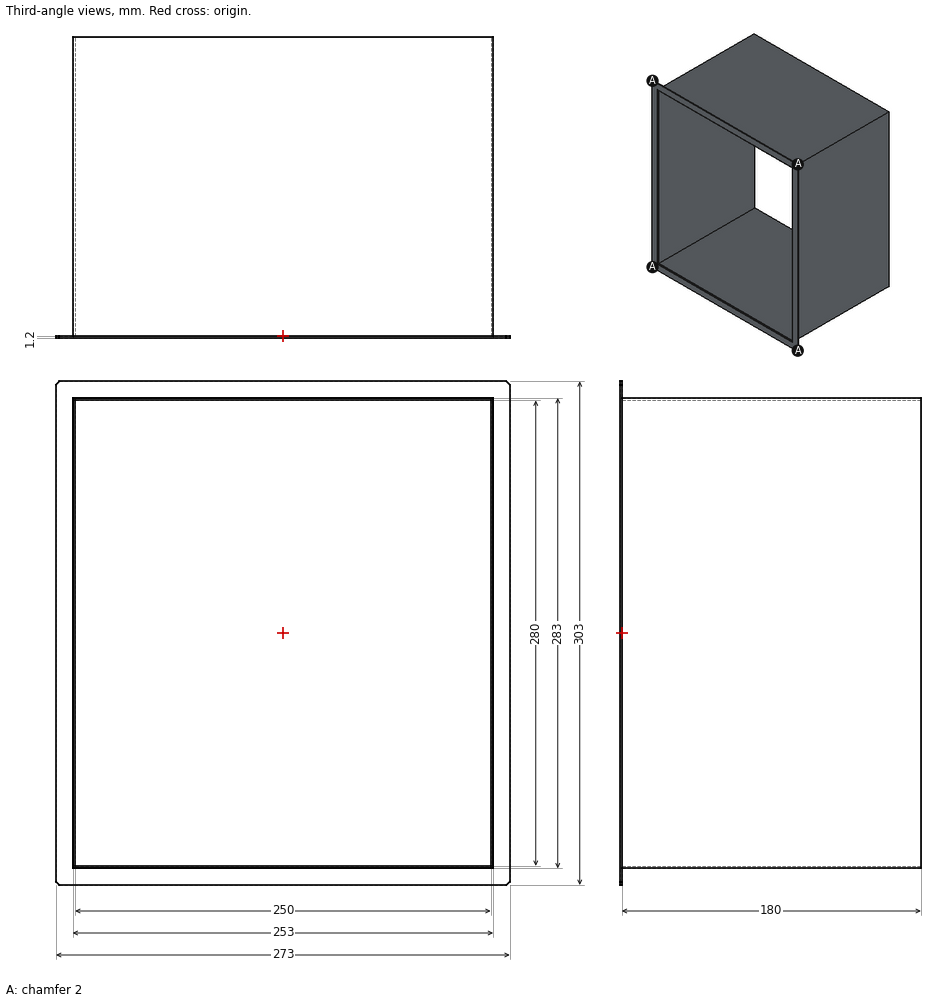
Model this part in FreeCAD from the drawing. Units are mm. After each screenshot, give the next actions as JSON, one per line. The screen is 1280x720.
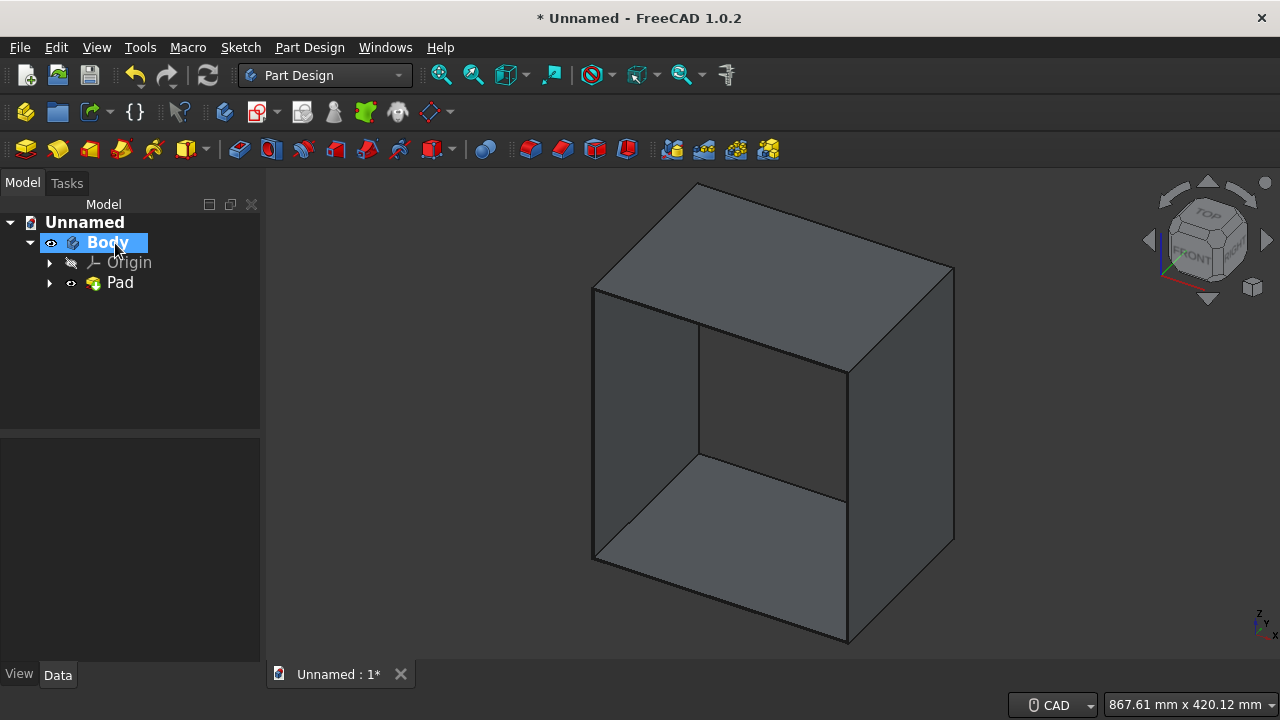
{"action": "left_click", "coordinate": [226, 112]}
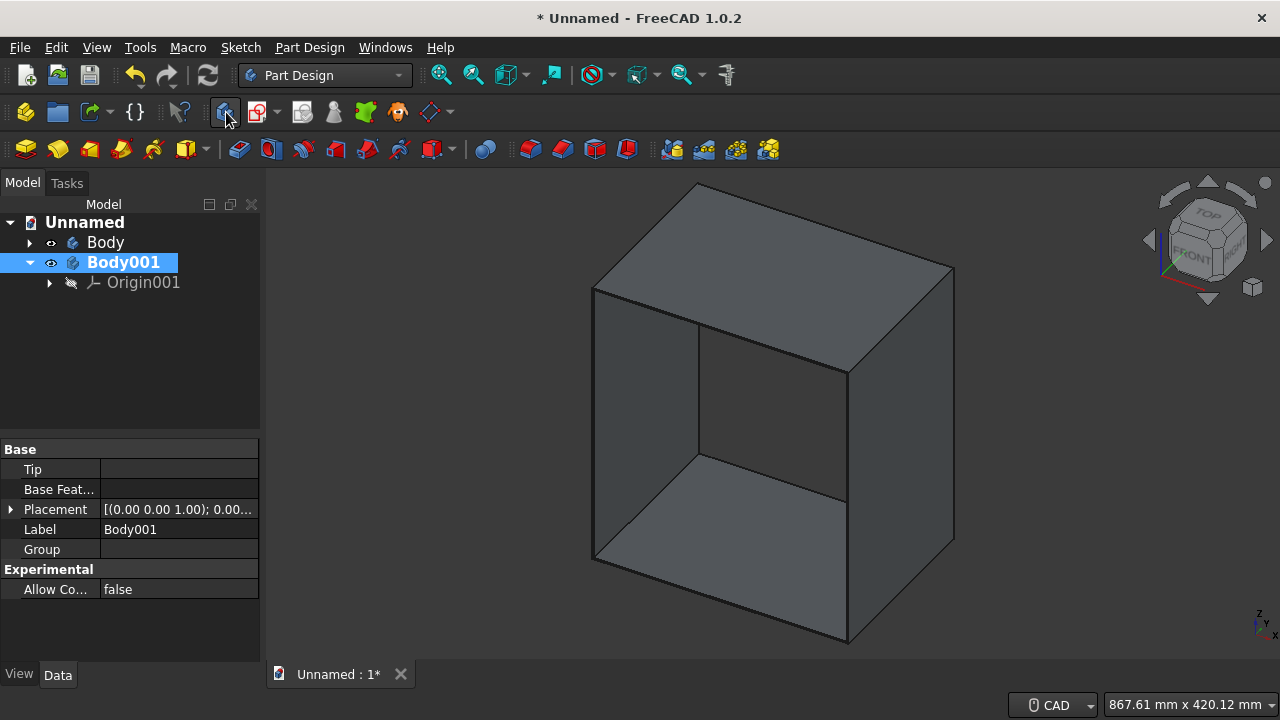
{"action": "left_click", "coordinate": [306, 619]}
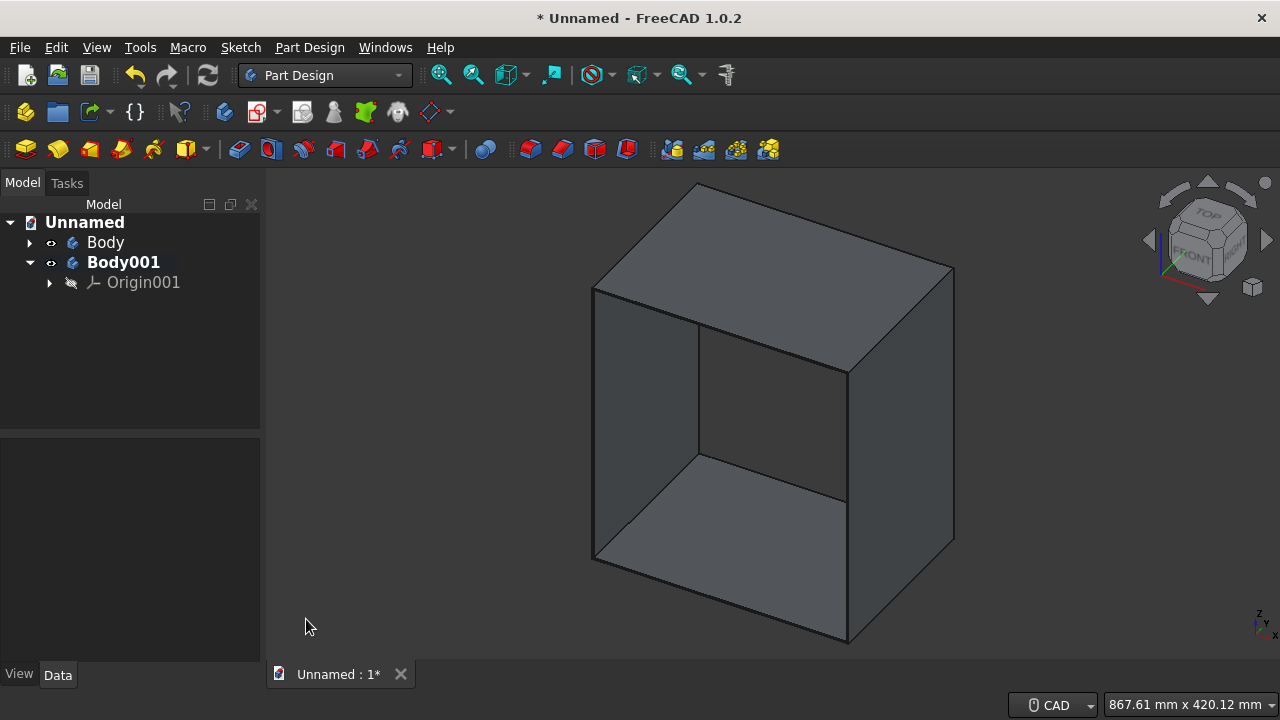
{"action": "left_click", "coordinate": [258, 112]}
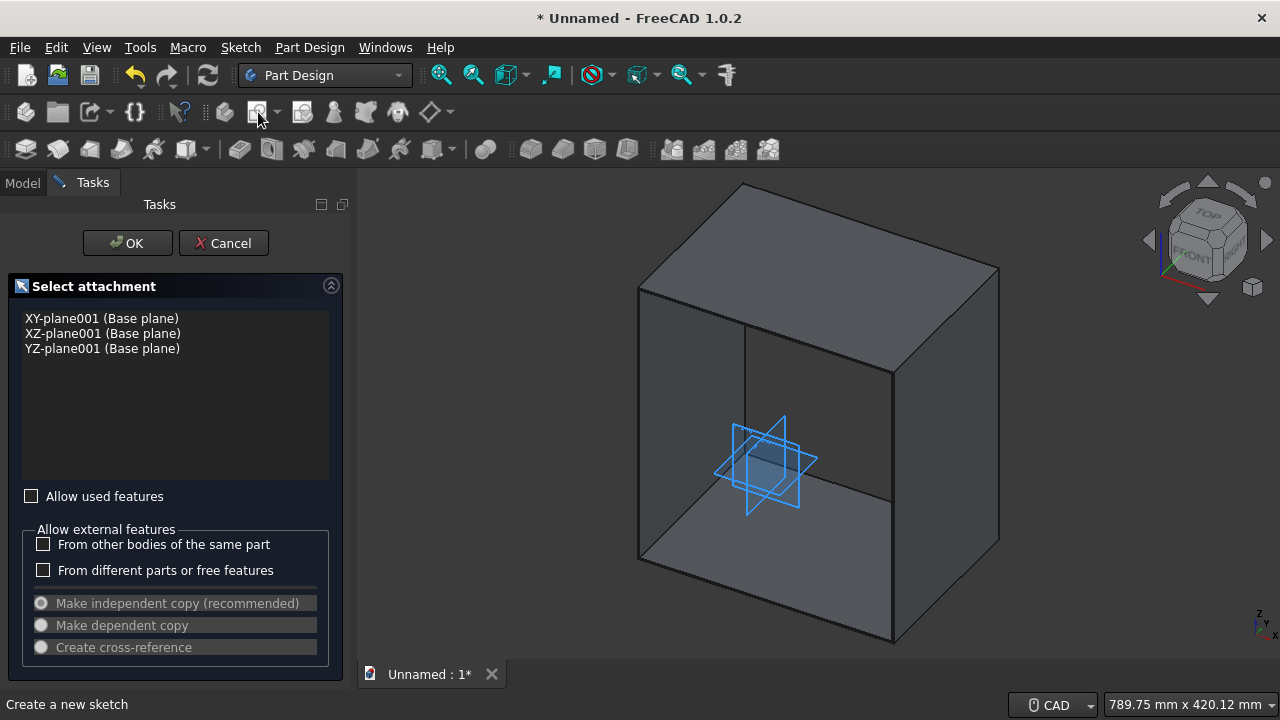
{"action": "left_click", "coordinate": [82, 334]}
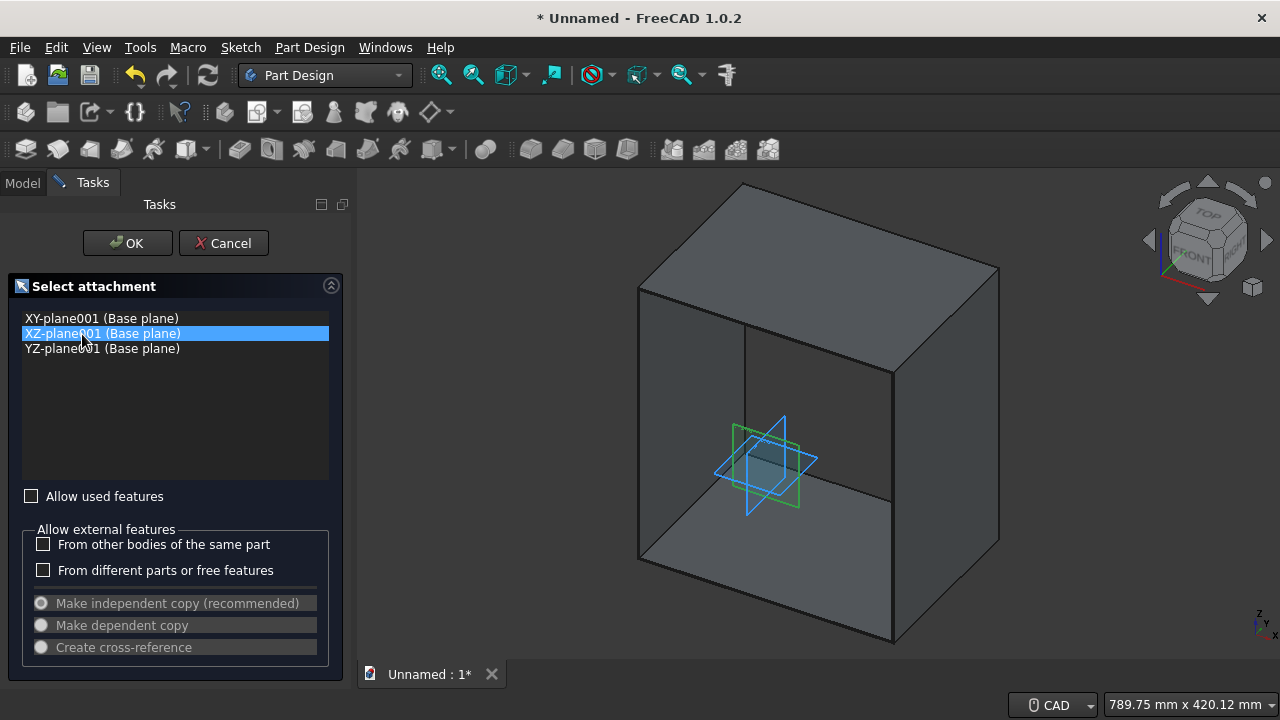
{"action": "left_click", "coordinate": [128, 243]}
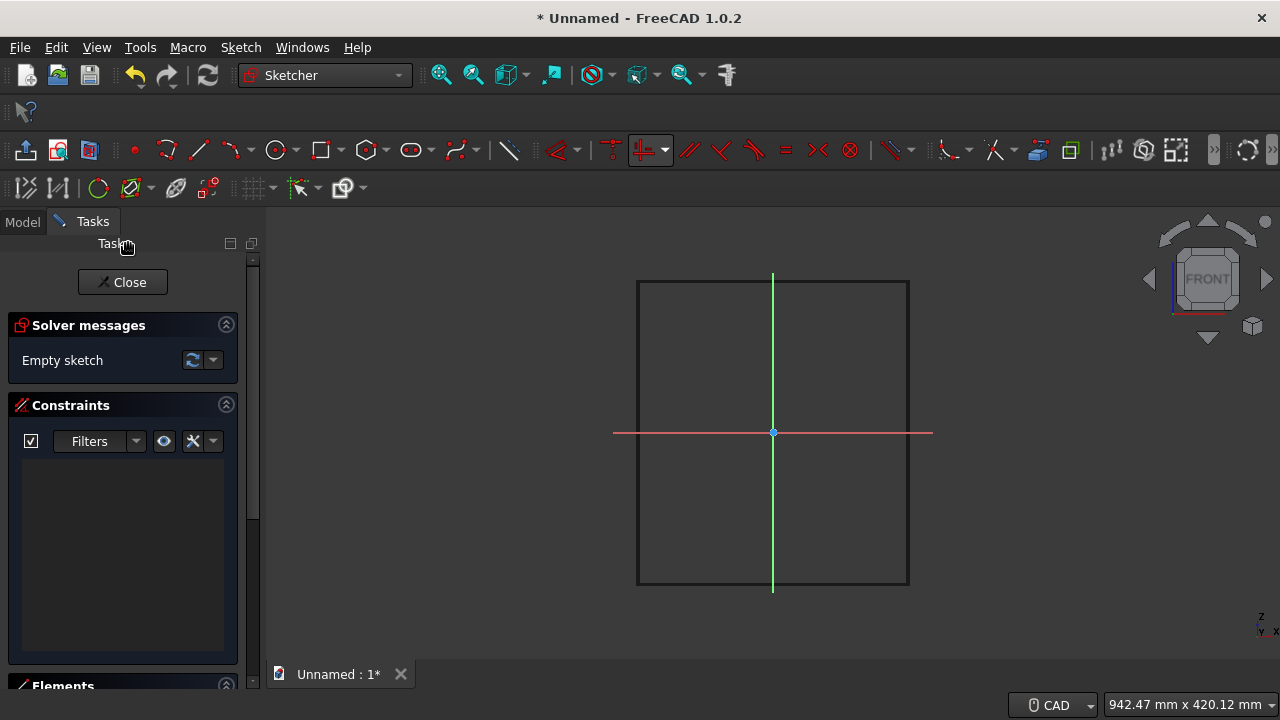
{"action": "key", "text": "g v"}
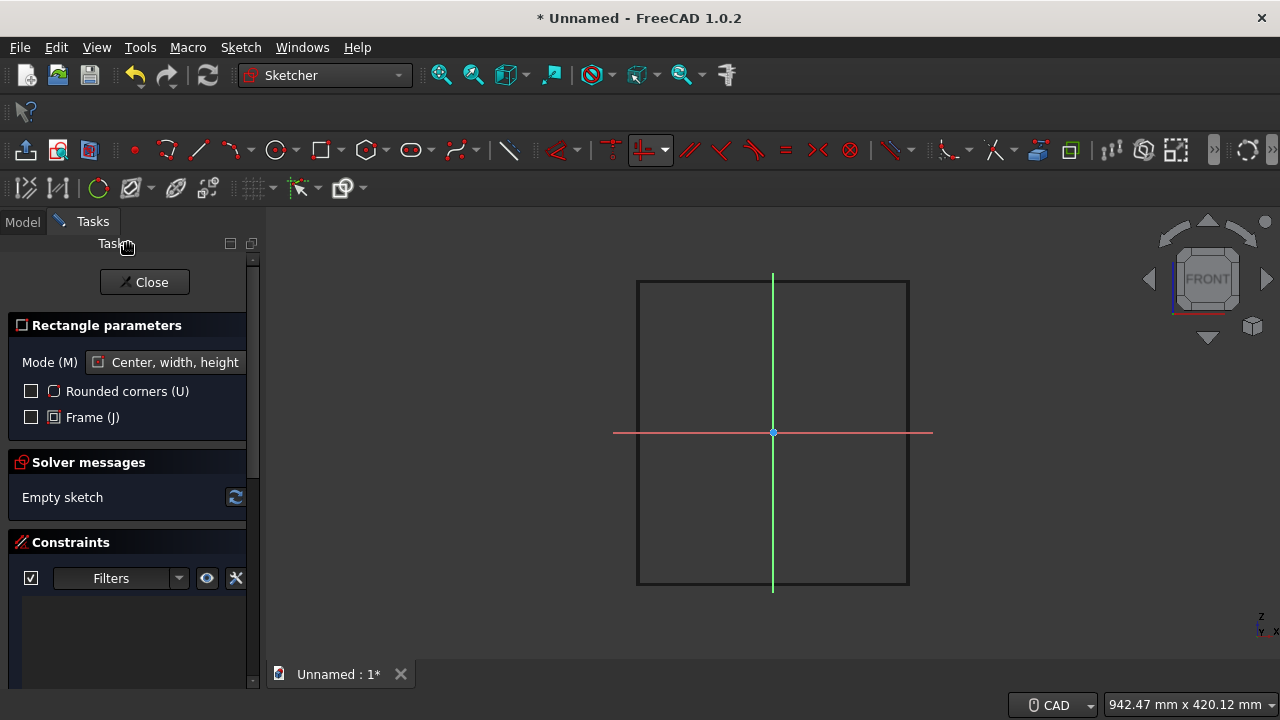
{"action": "left_click", "coordinate": [773, 433]}
{"action": "left_click", "coordinate": [920, 270]}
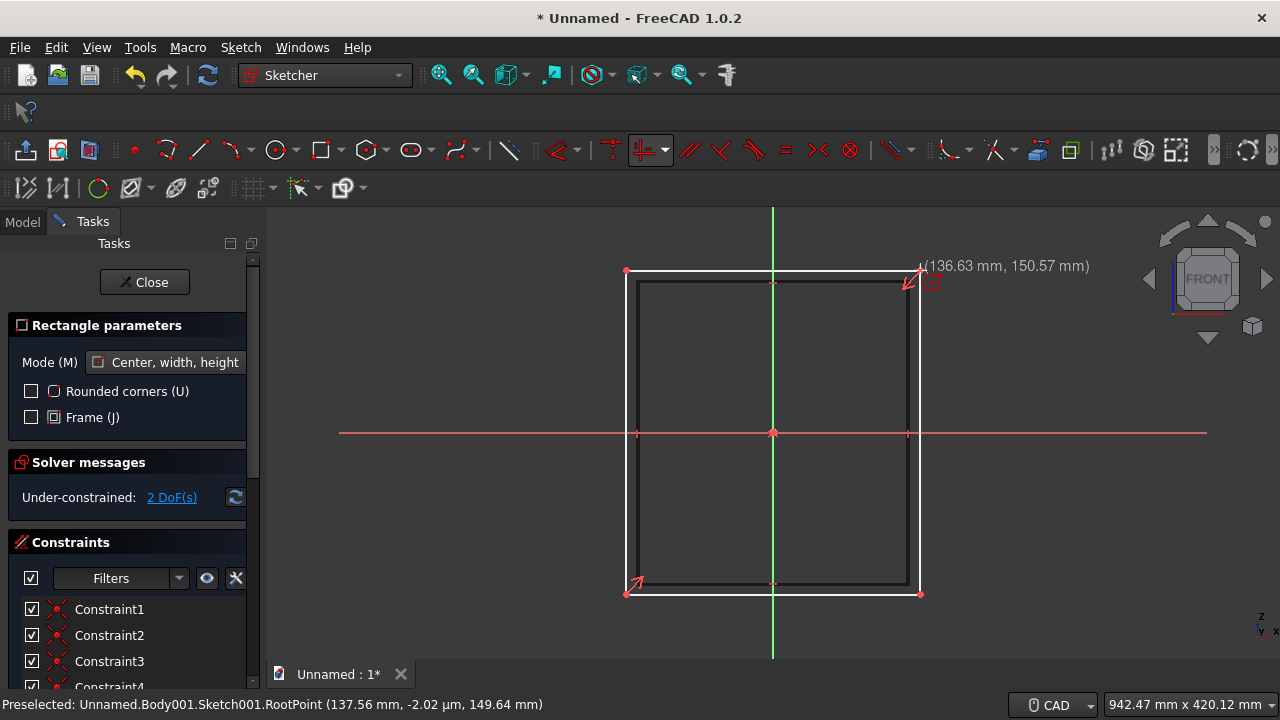
{"action": "left_click", "coordinate": [773, 433]}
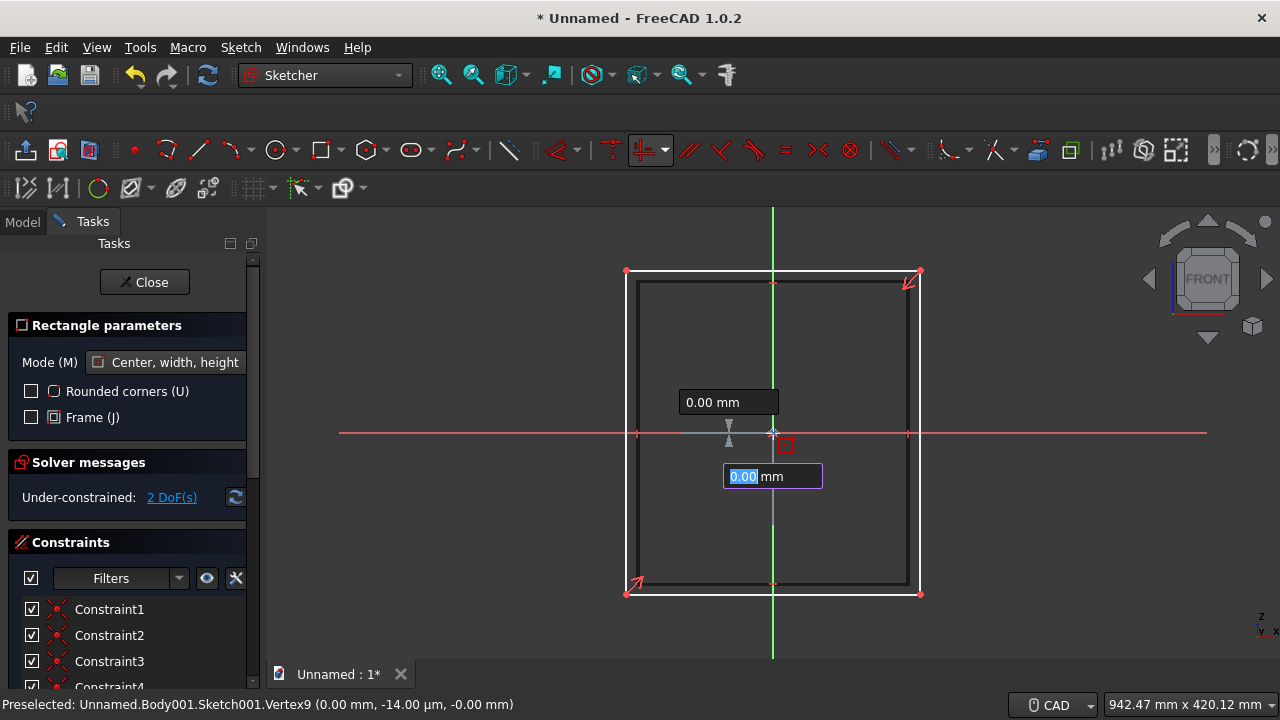
{"action": "scroll", "coordinate": [909, 281], "scroll_direction": "up", "scroll_amount": 2}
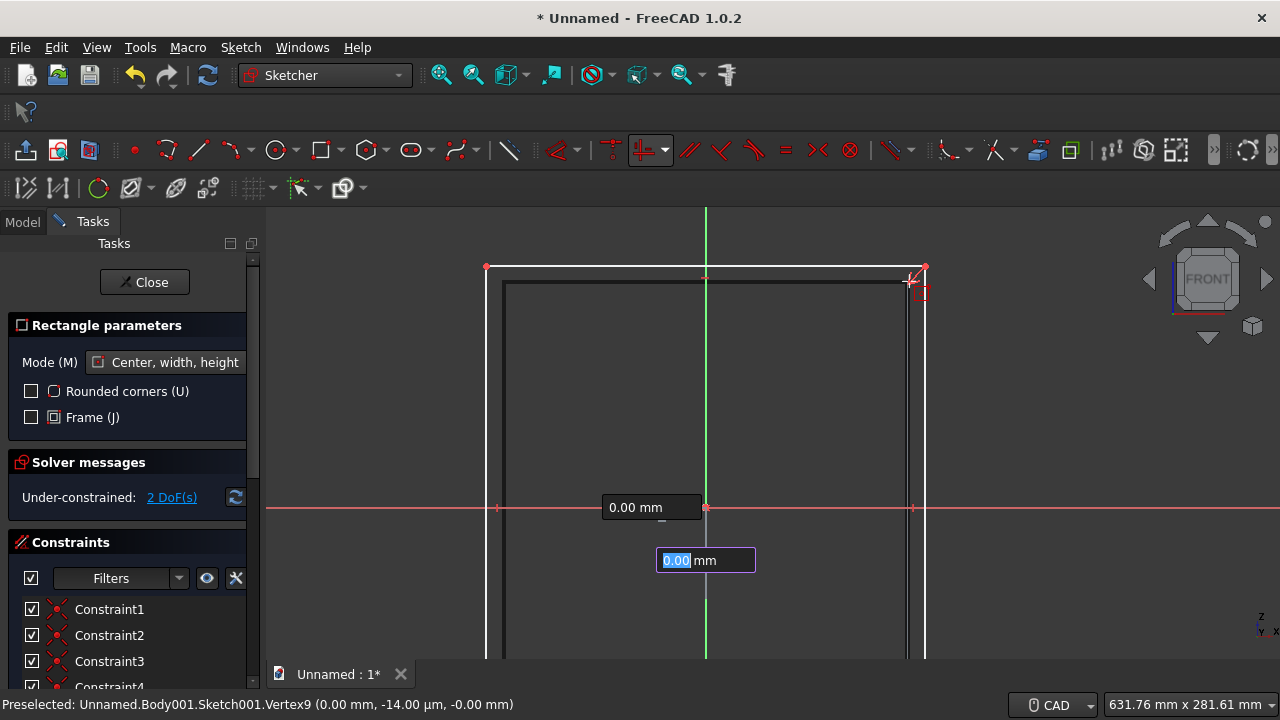
{"action": "left_click", "coordinate": [909, 281]}
{"action": "key", "text": "Escape"}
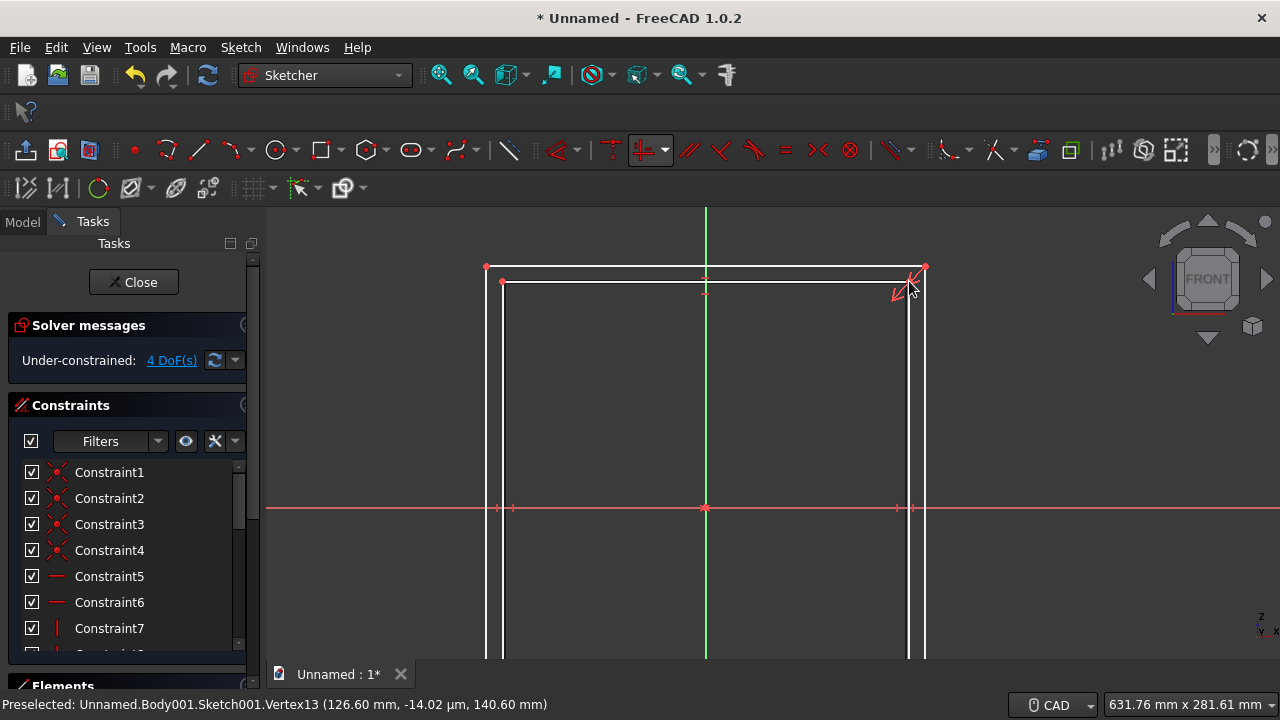
{"action": "key", "text": "d"}